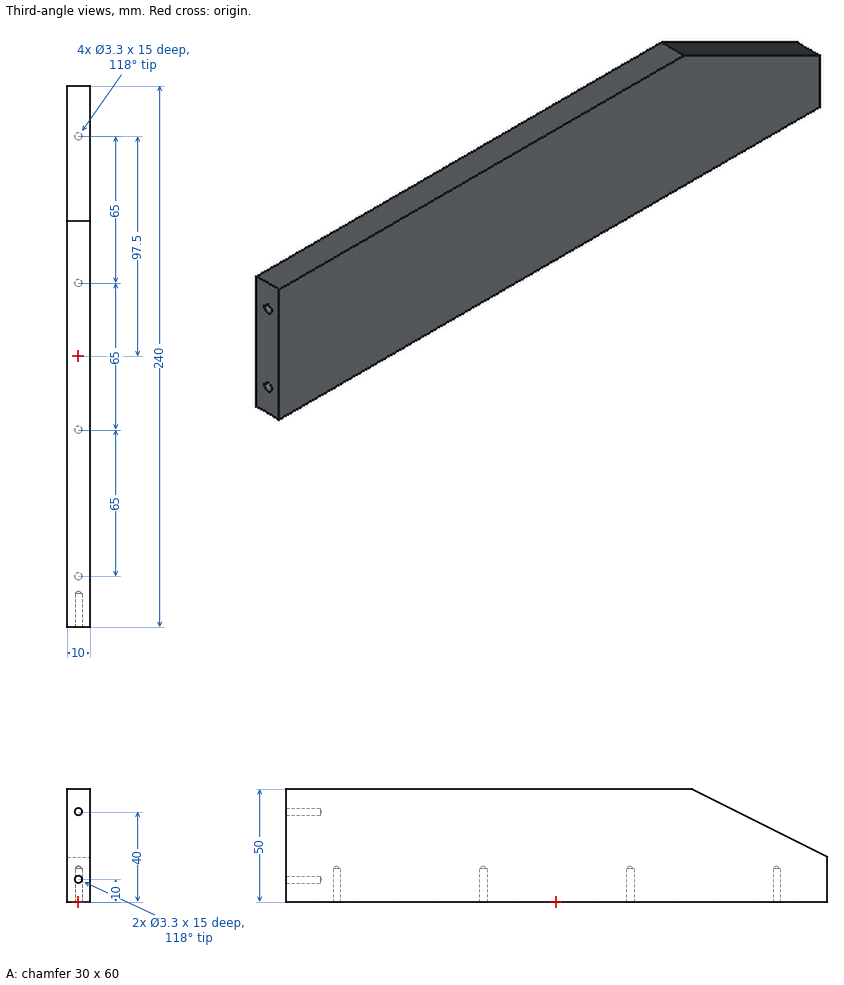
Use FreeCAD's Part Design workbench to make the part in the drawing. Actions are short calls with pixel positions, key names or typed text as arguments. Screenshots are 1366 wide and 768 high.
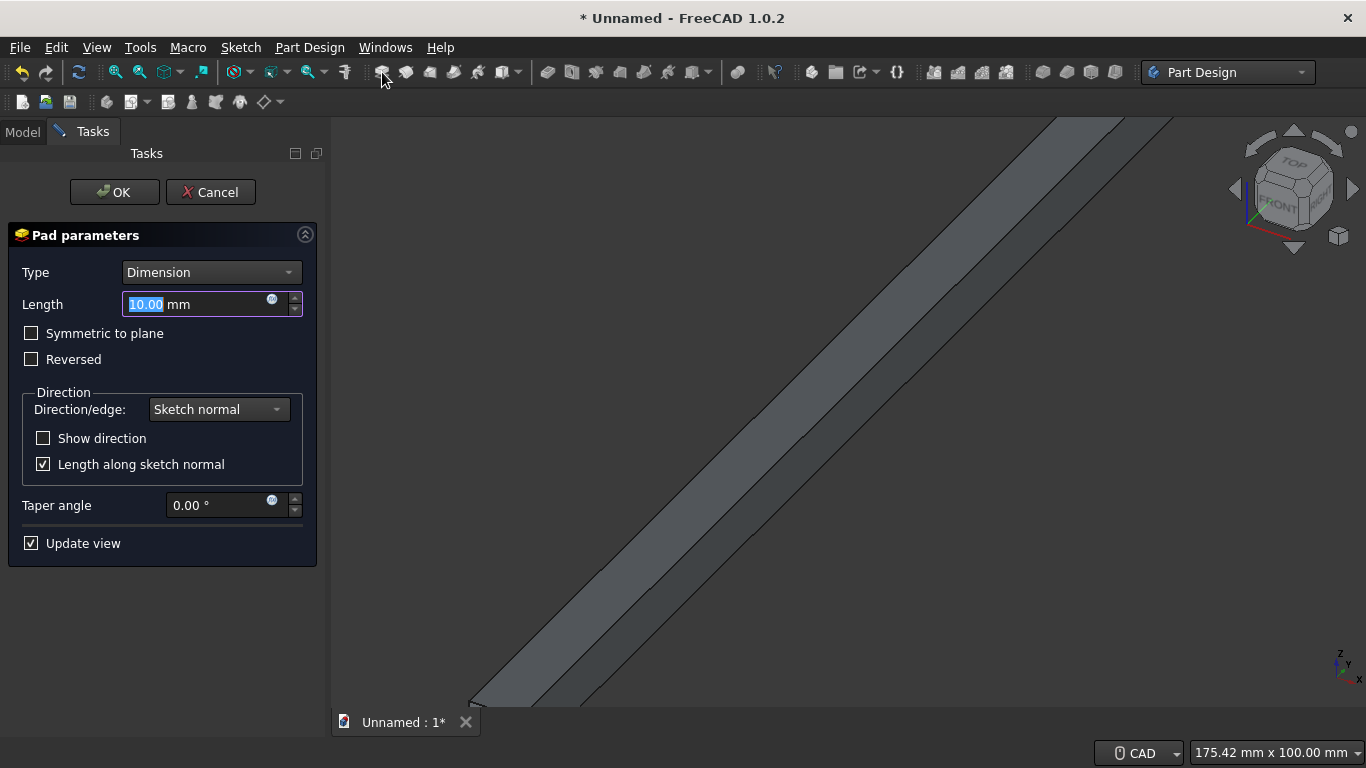
text(50)
key(Tab)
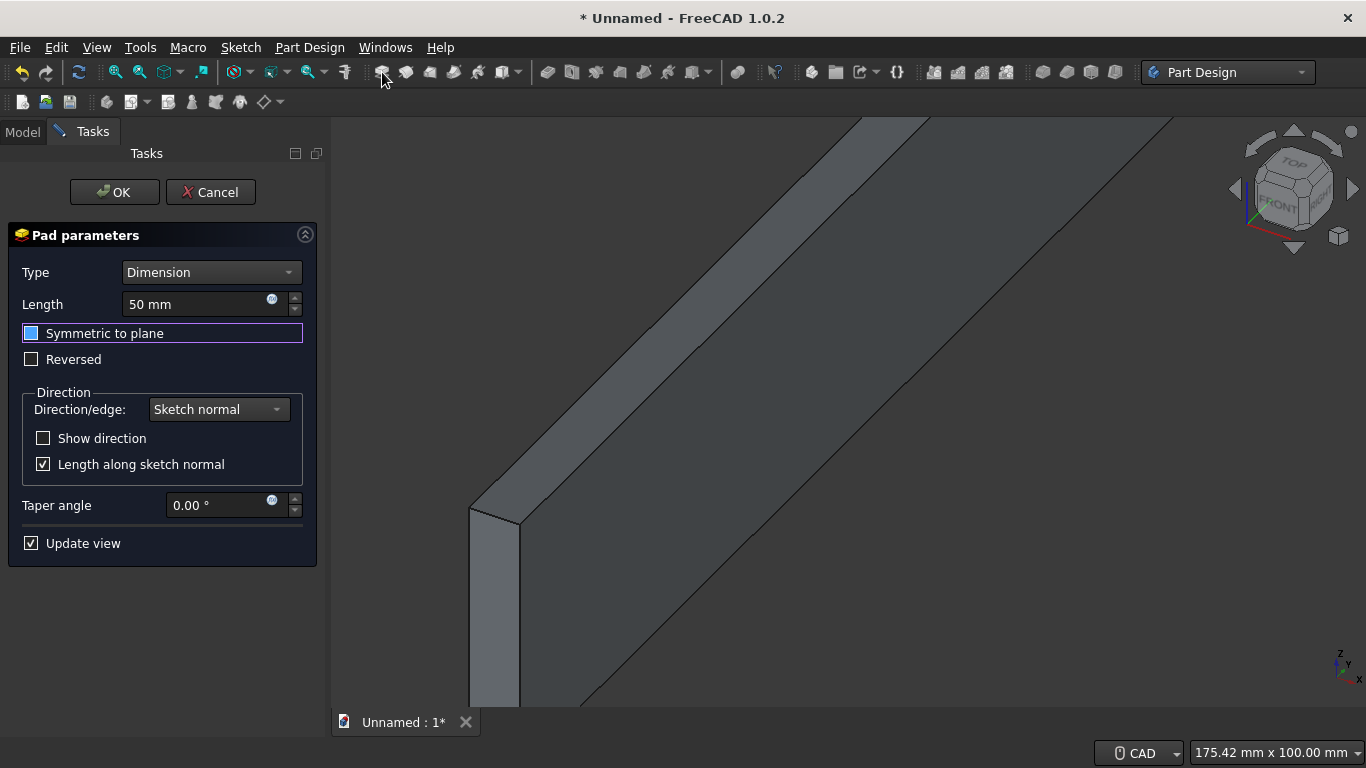
click(115, 192)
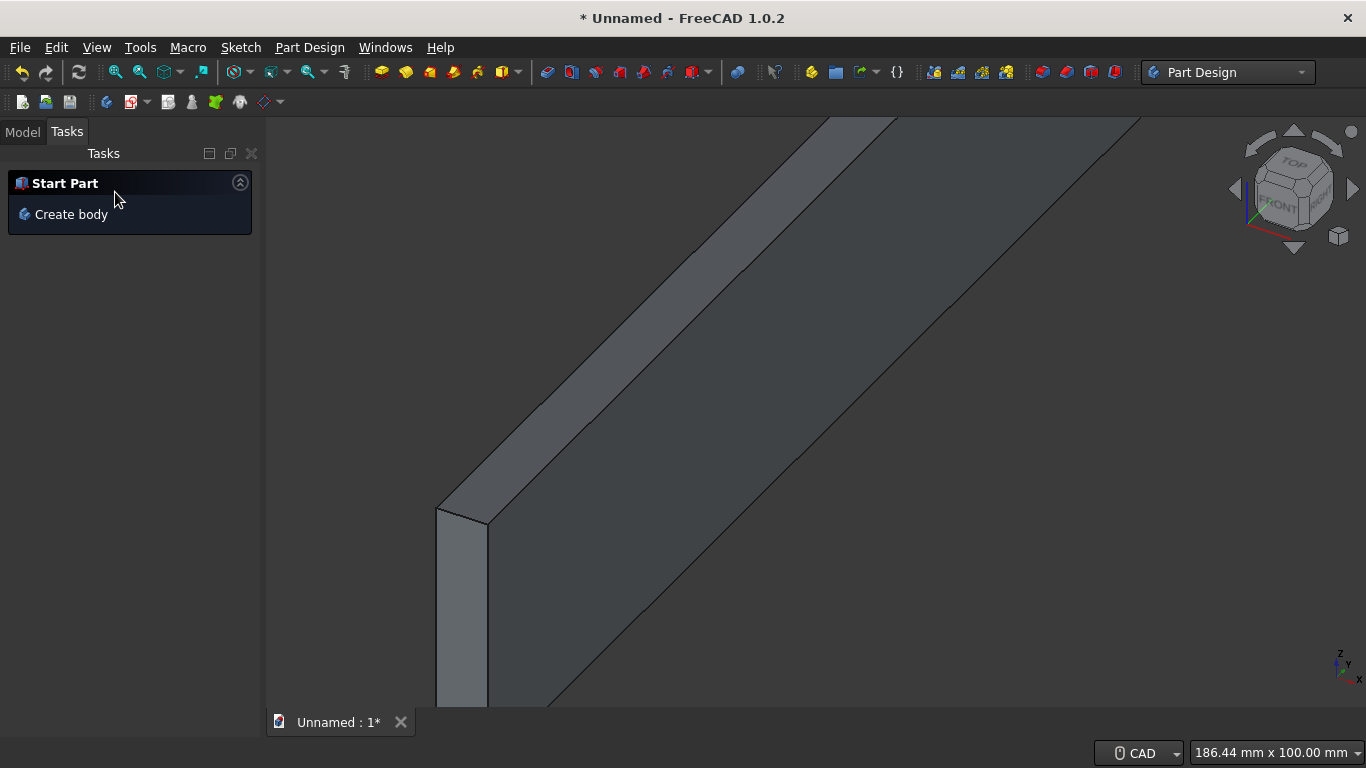
click(116, 72)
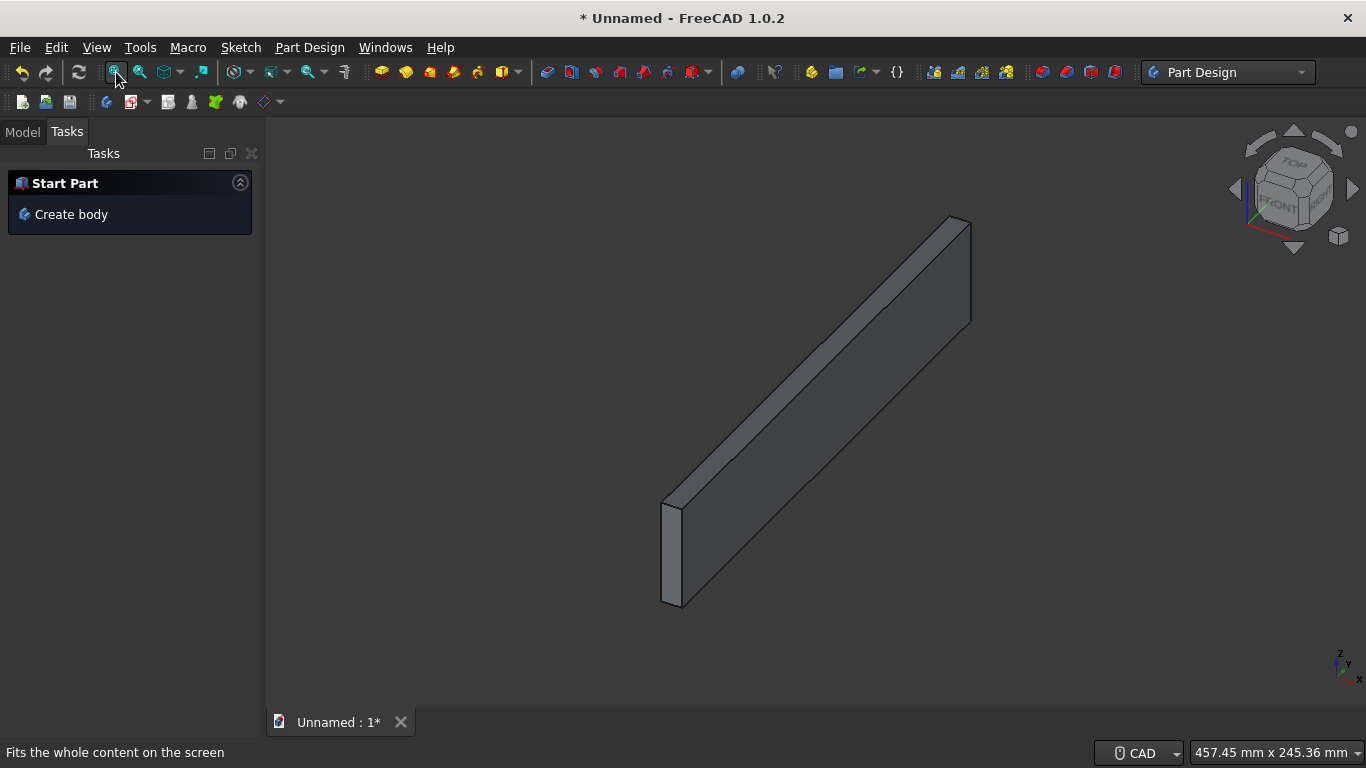
click(132, 102)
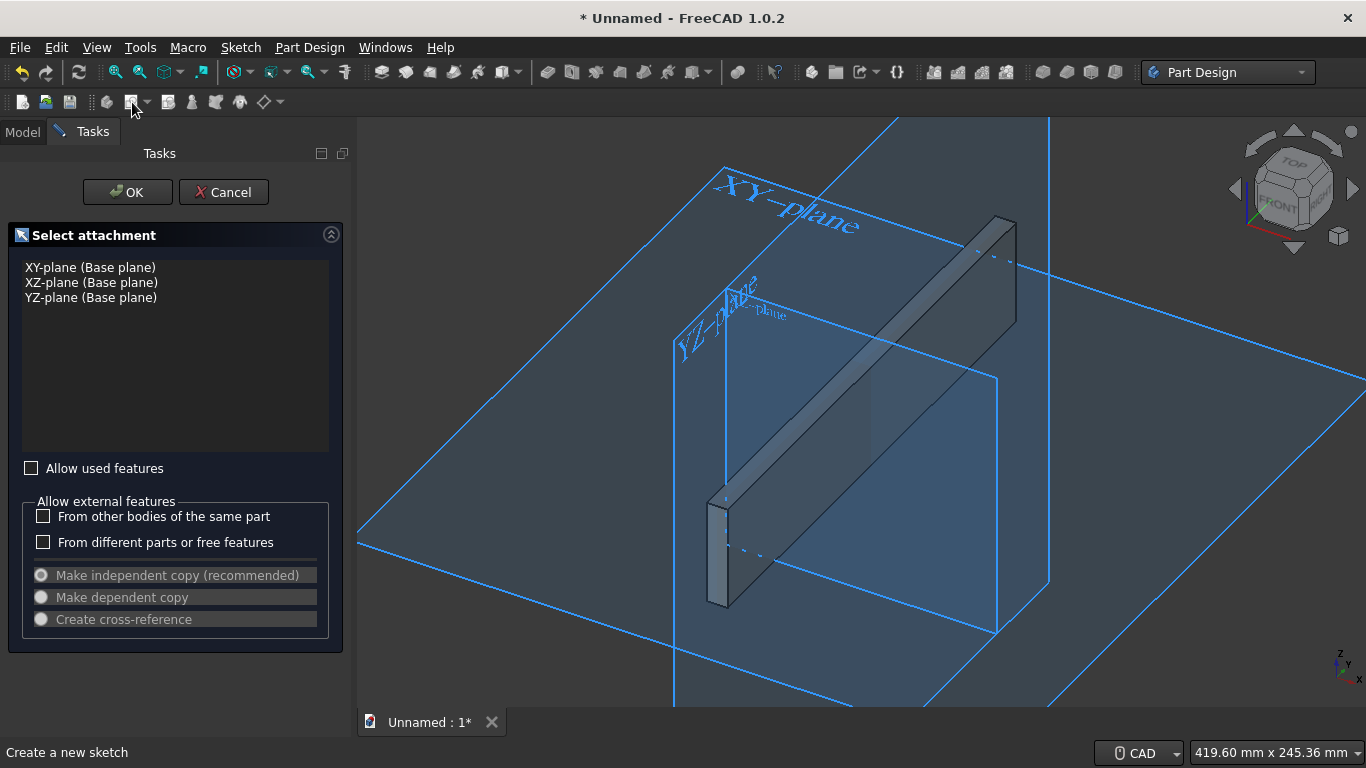
click(82, 268)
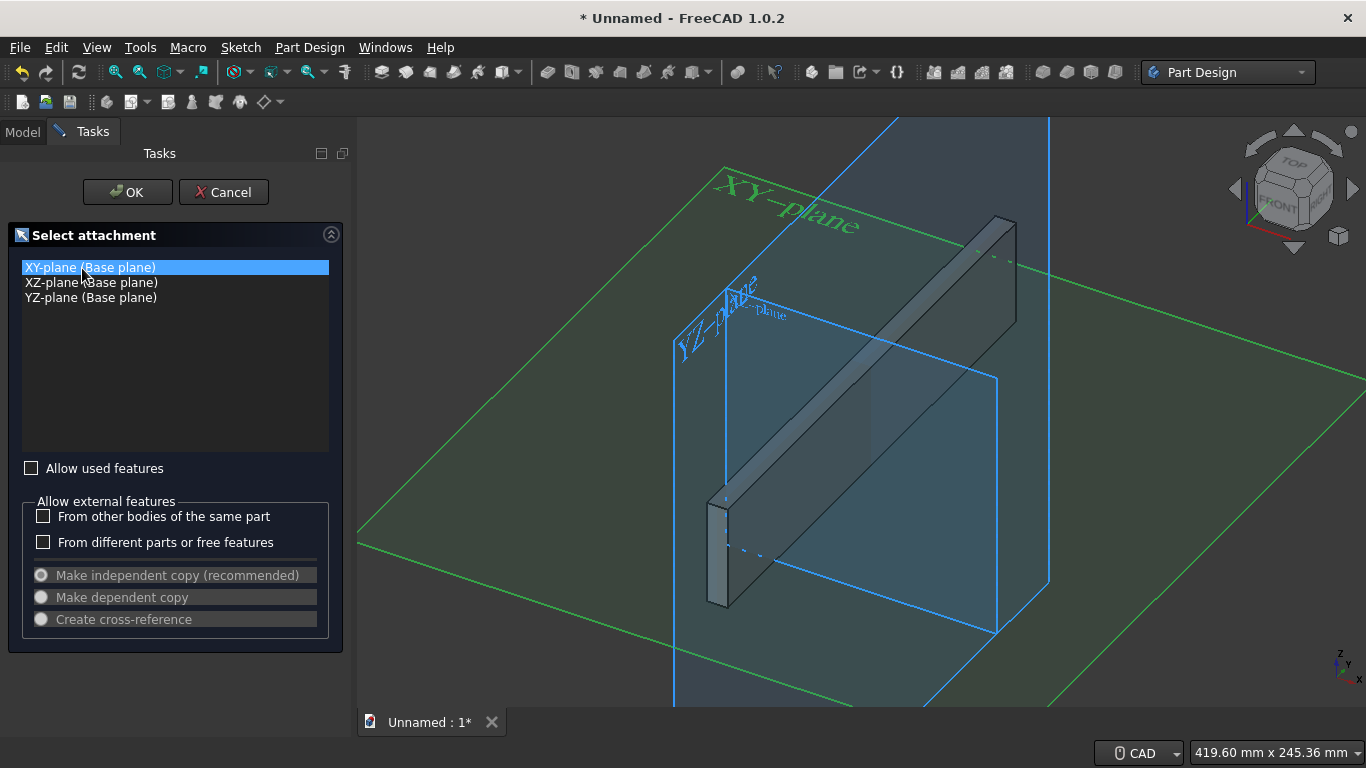
click(128, 192)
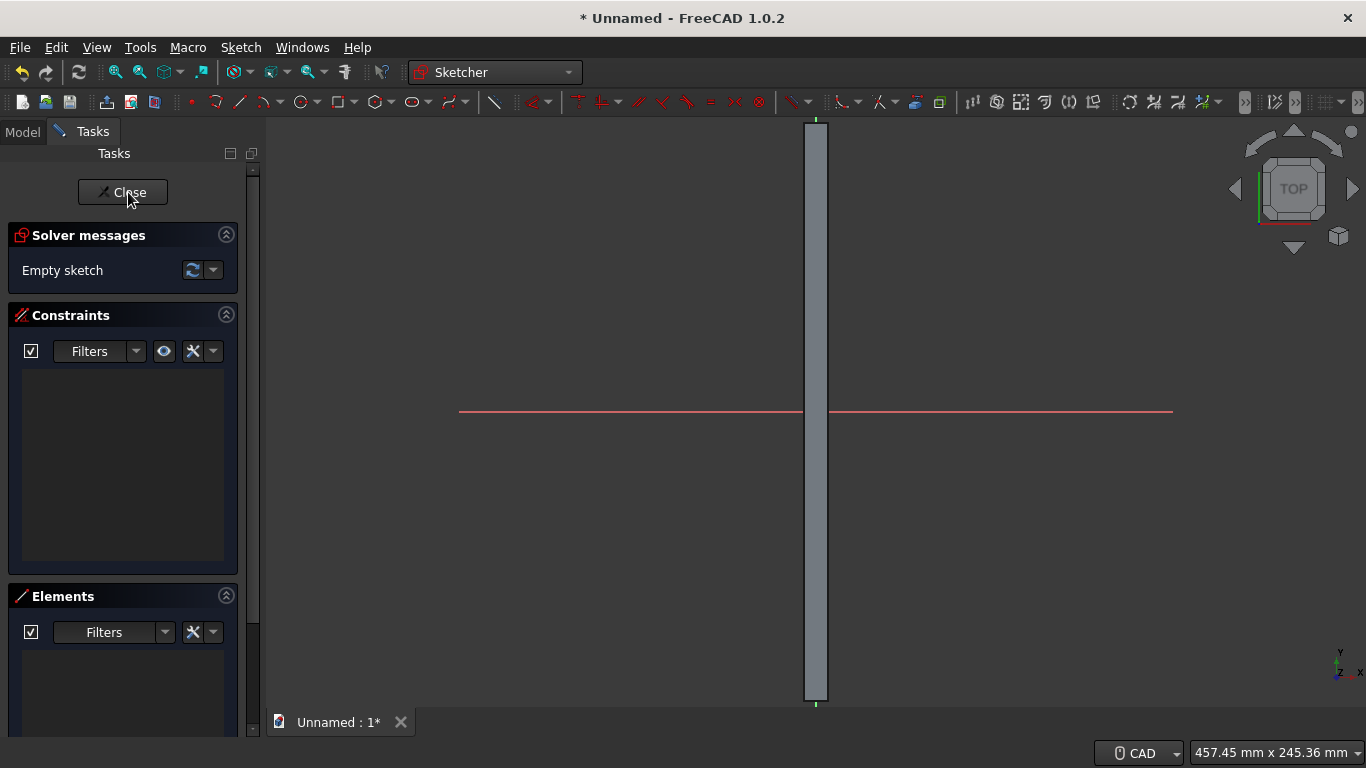
key(q)
key(s)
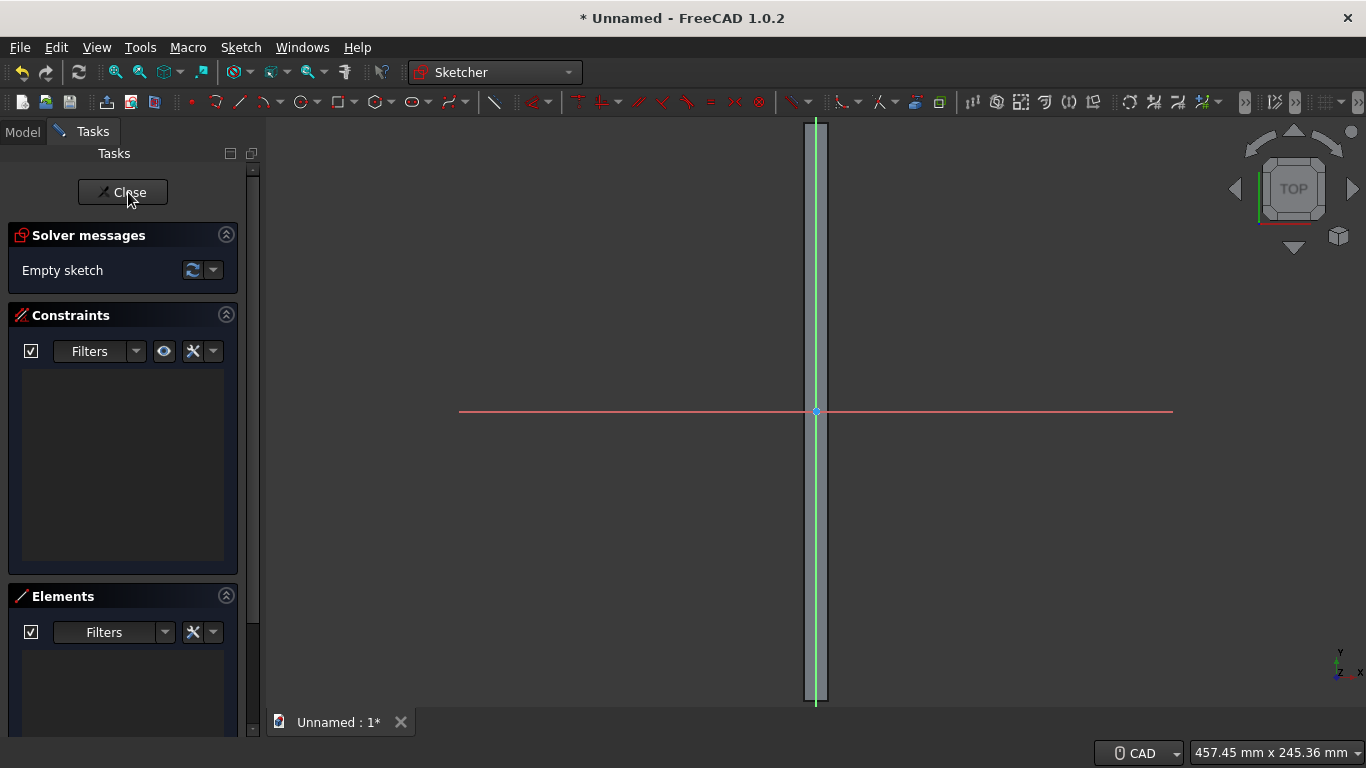
key(g)
key(c)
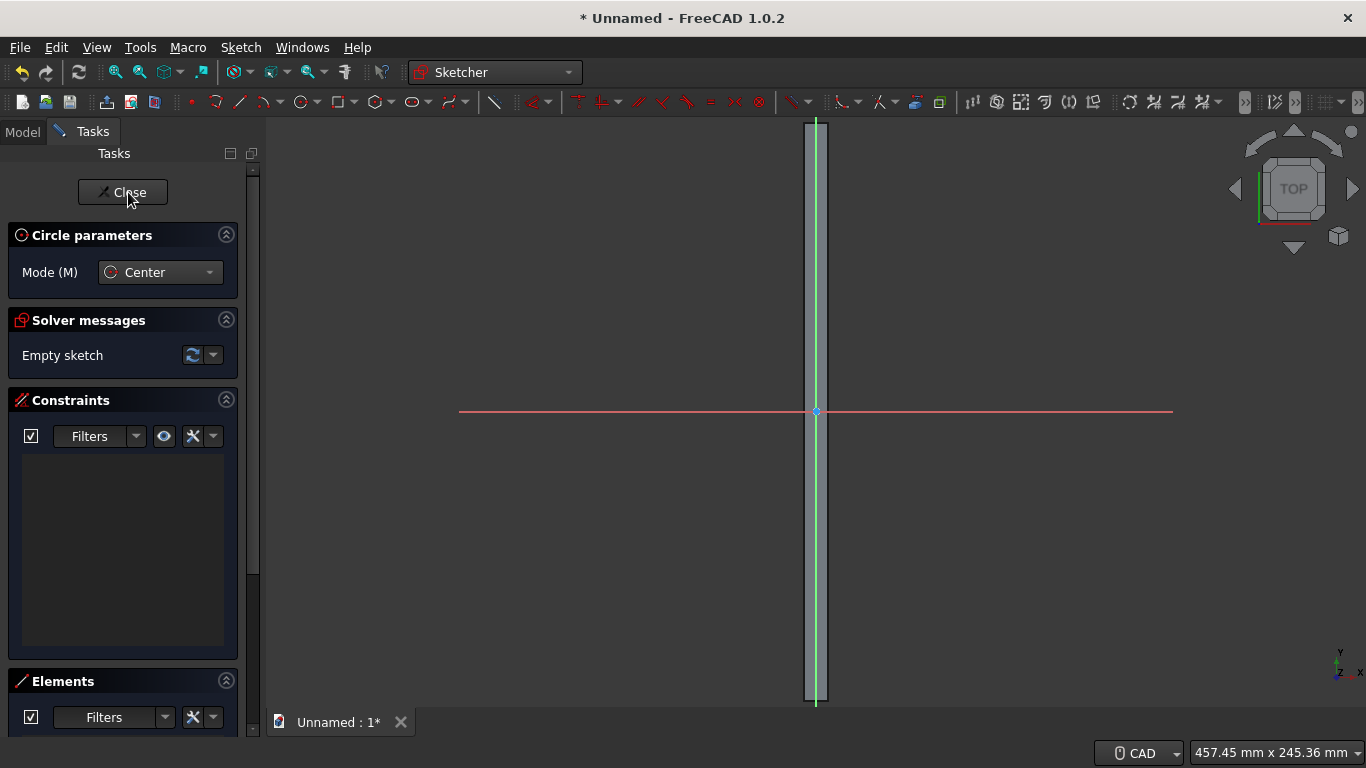
scroll(816, 178, up, 9)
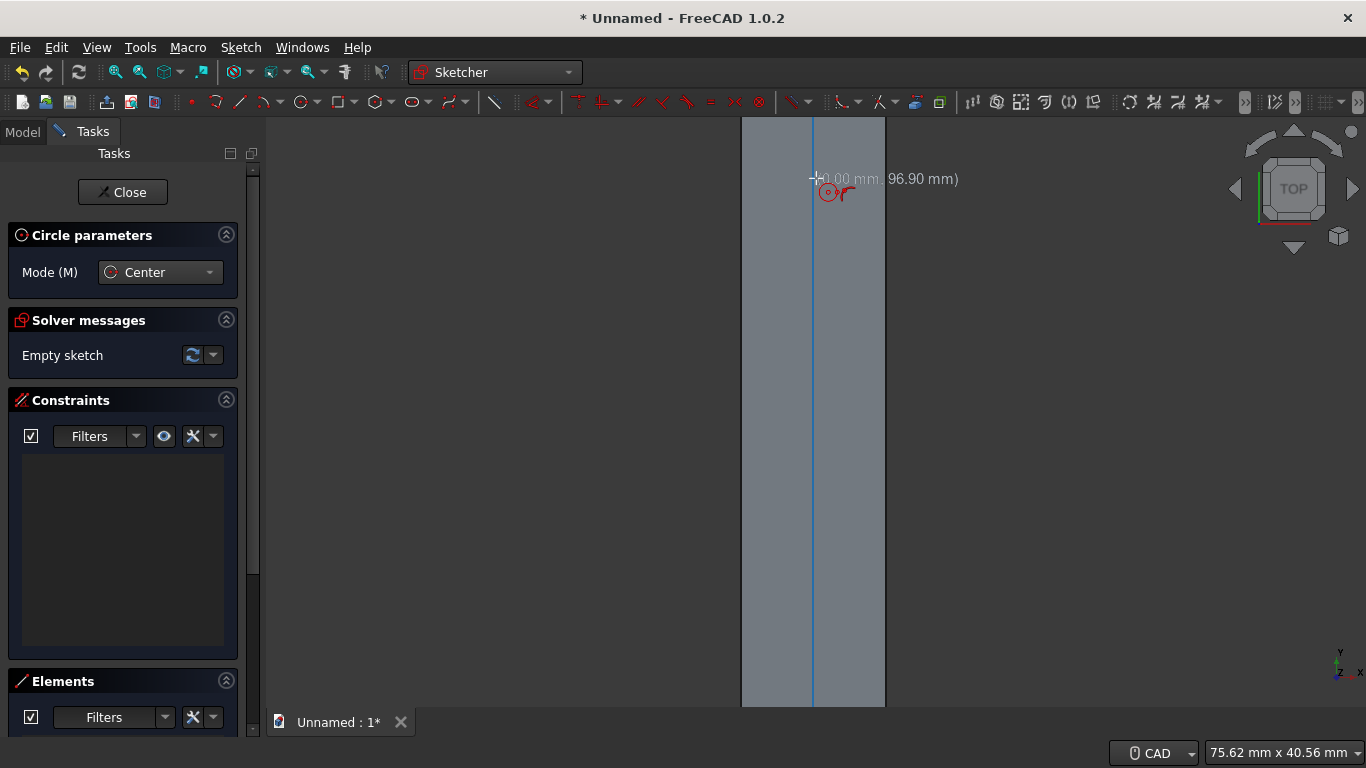
scroll(737, 227, down, 10)